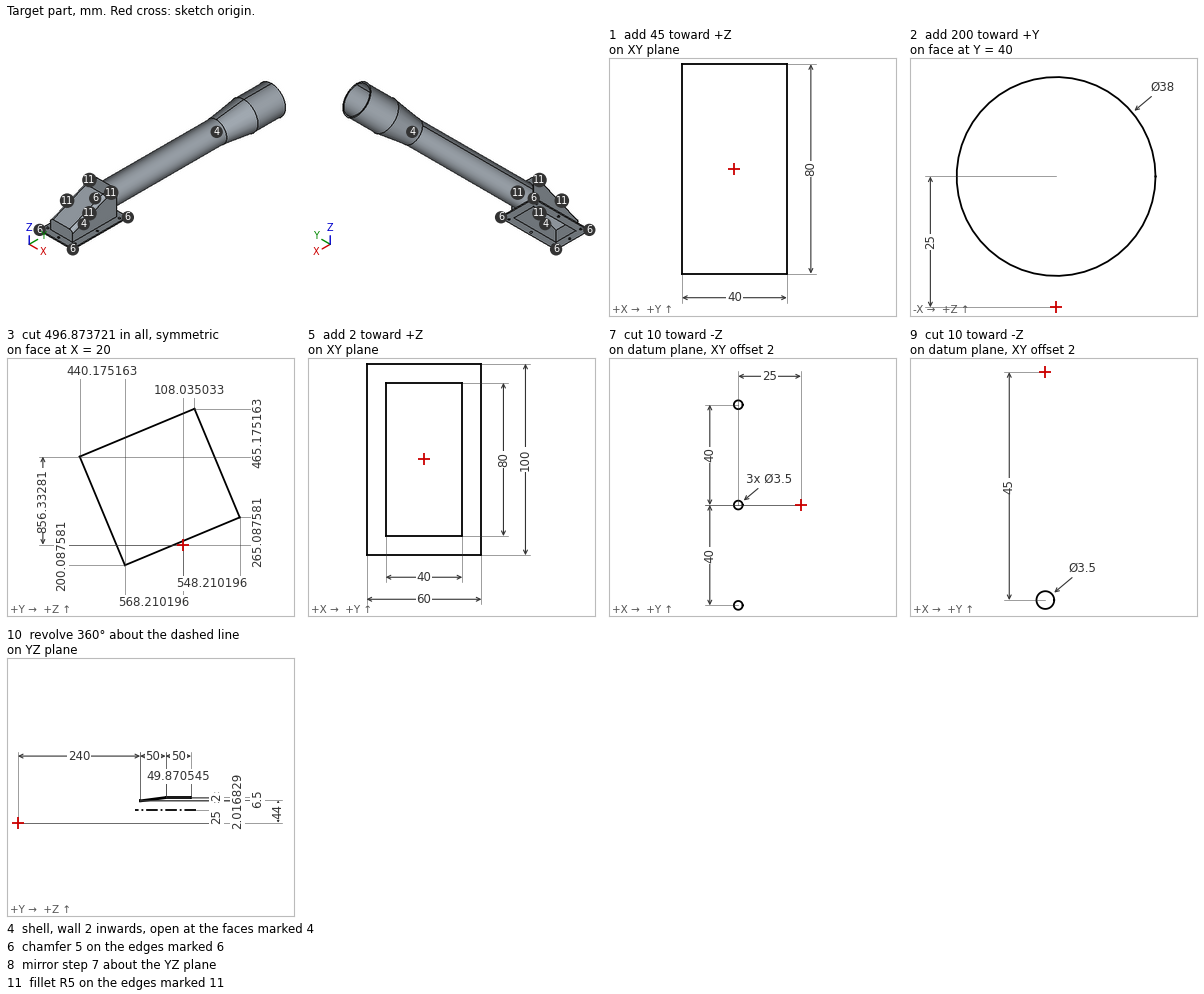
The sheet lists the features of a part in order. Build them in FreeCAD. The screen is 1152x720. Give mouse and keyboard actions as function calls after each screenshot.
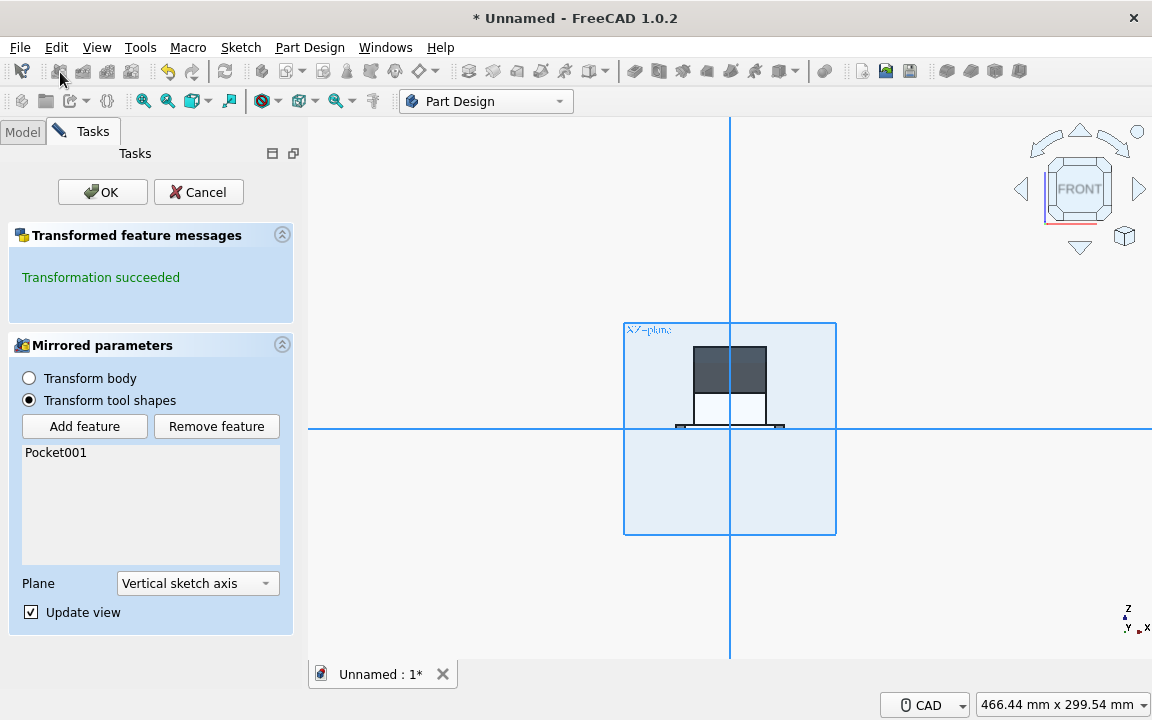
click(198, 584)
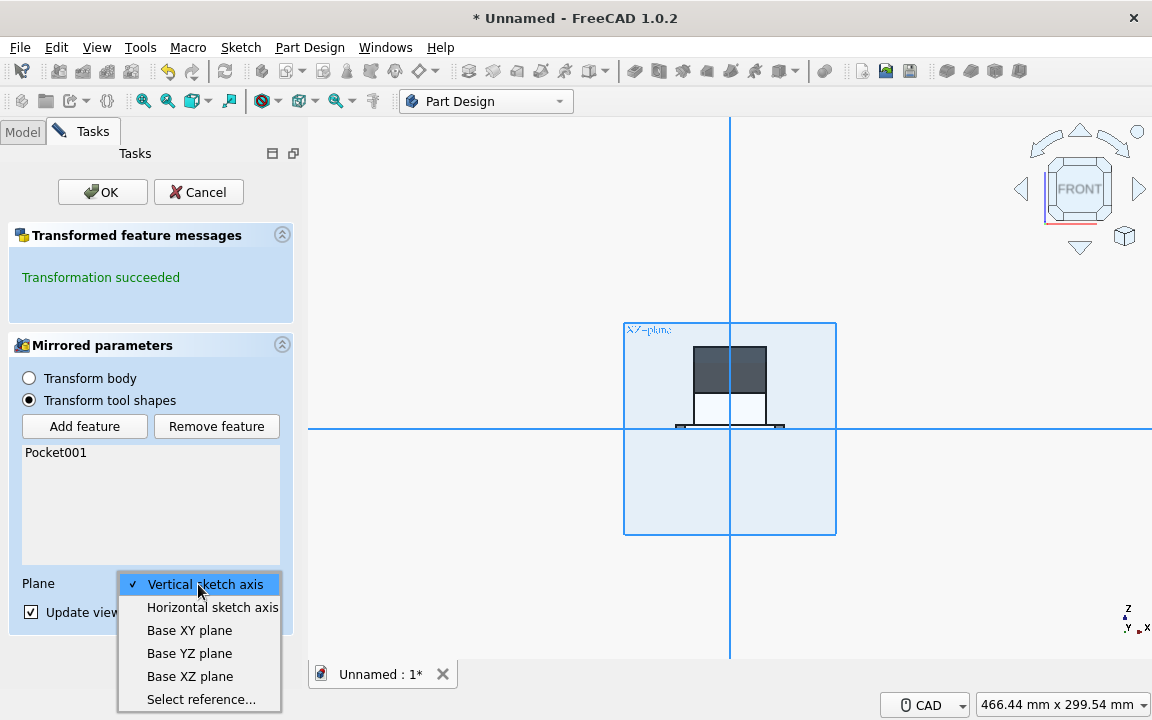
click(198, 654)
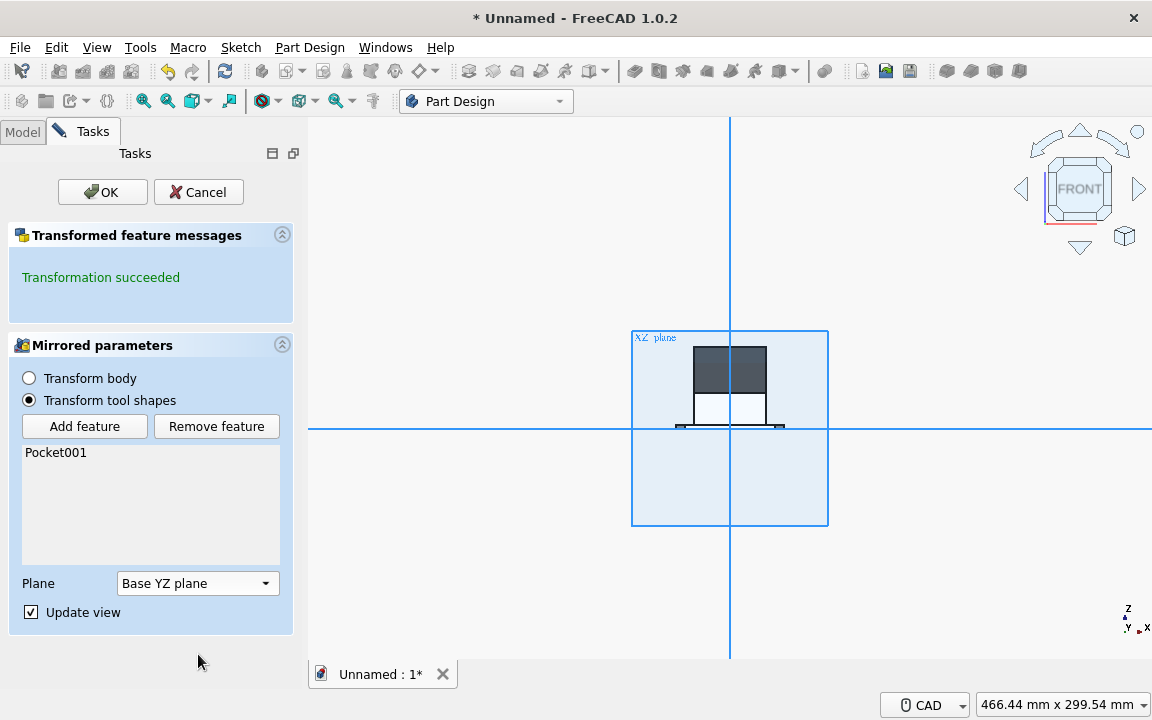
click(103, 192)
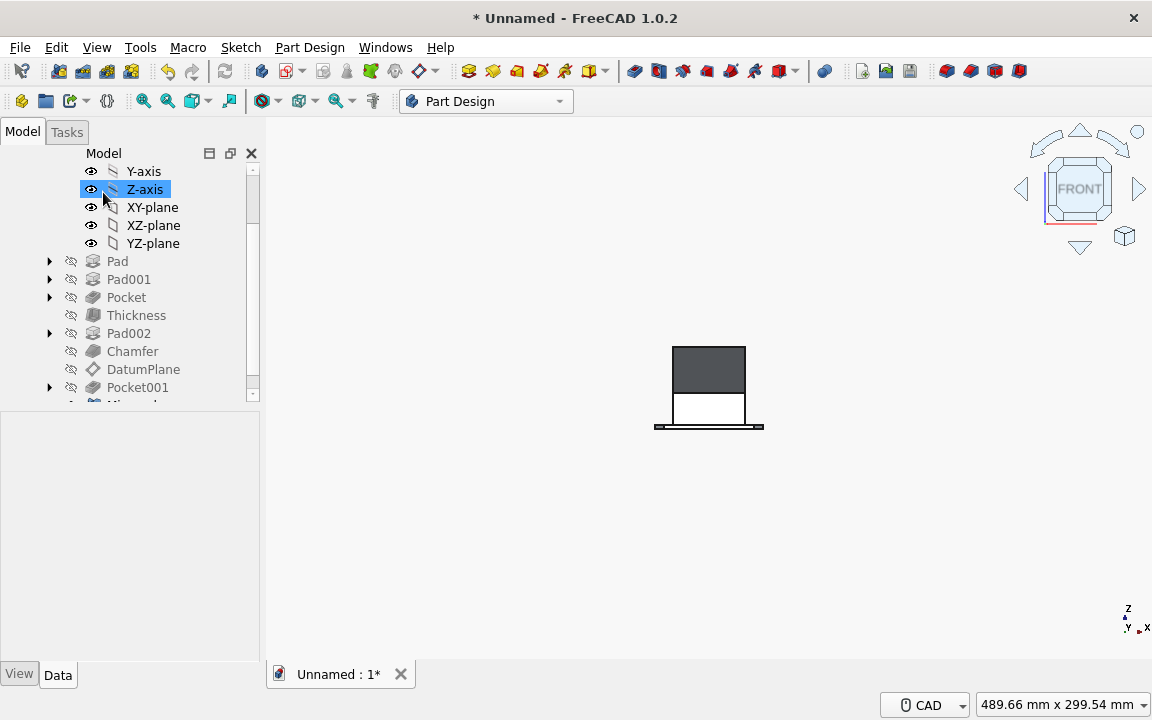
key(v)
key(f)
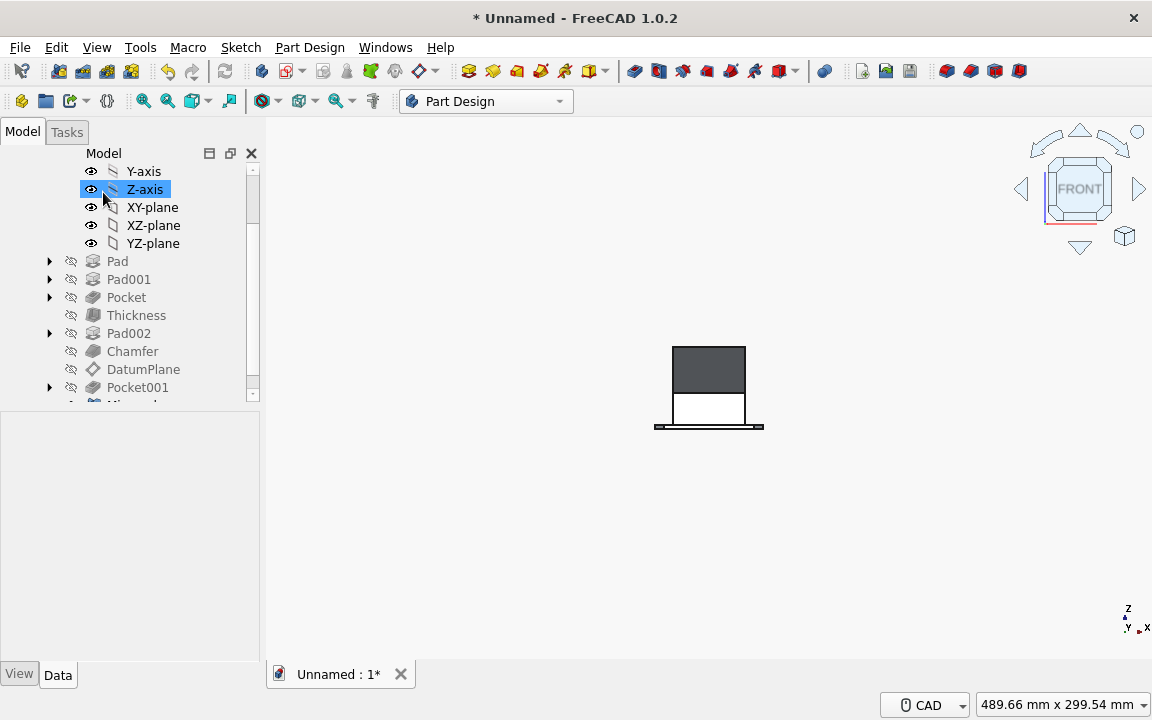
key(0)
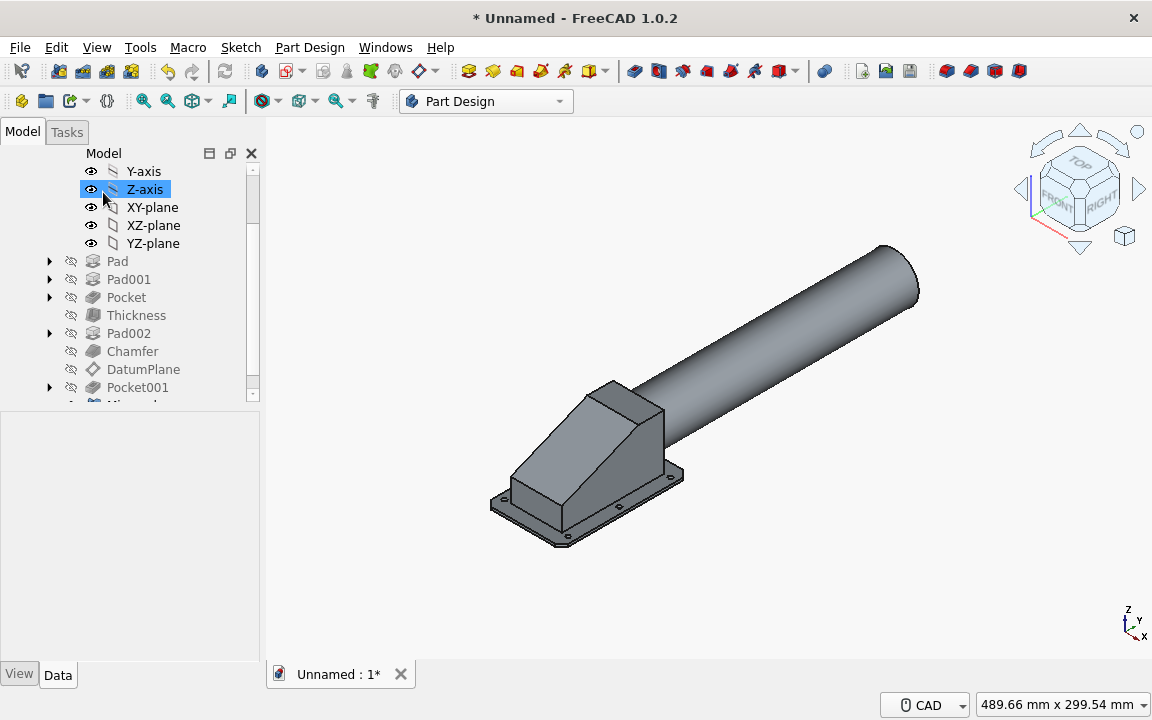
key(2)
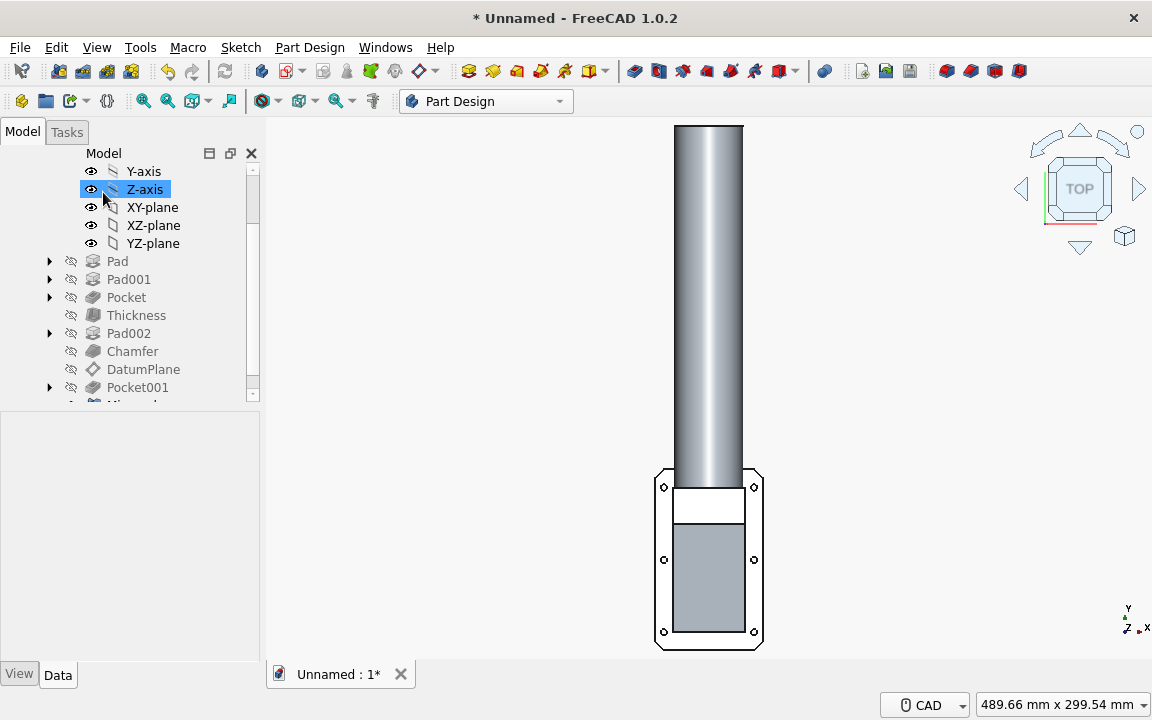
key(1)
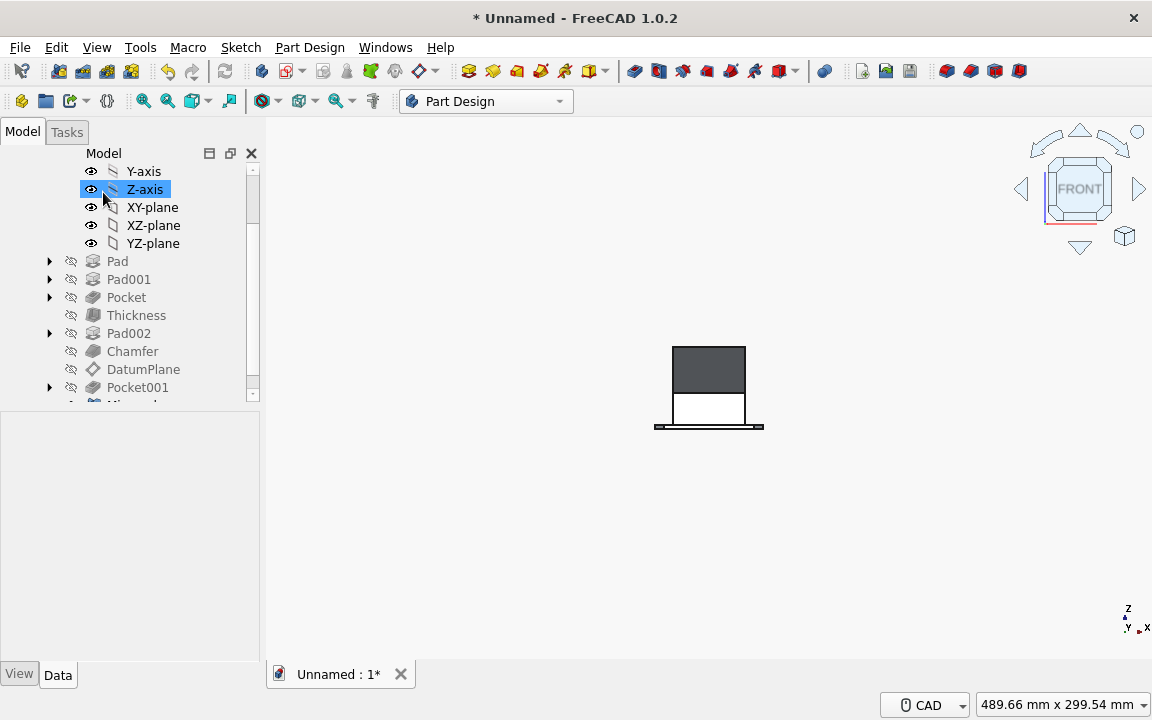
key(v)
key(f)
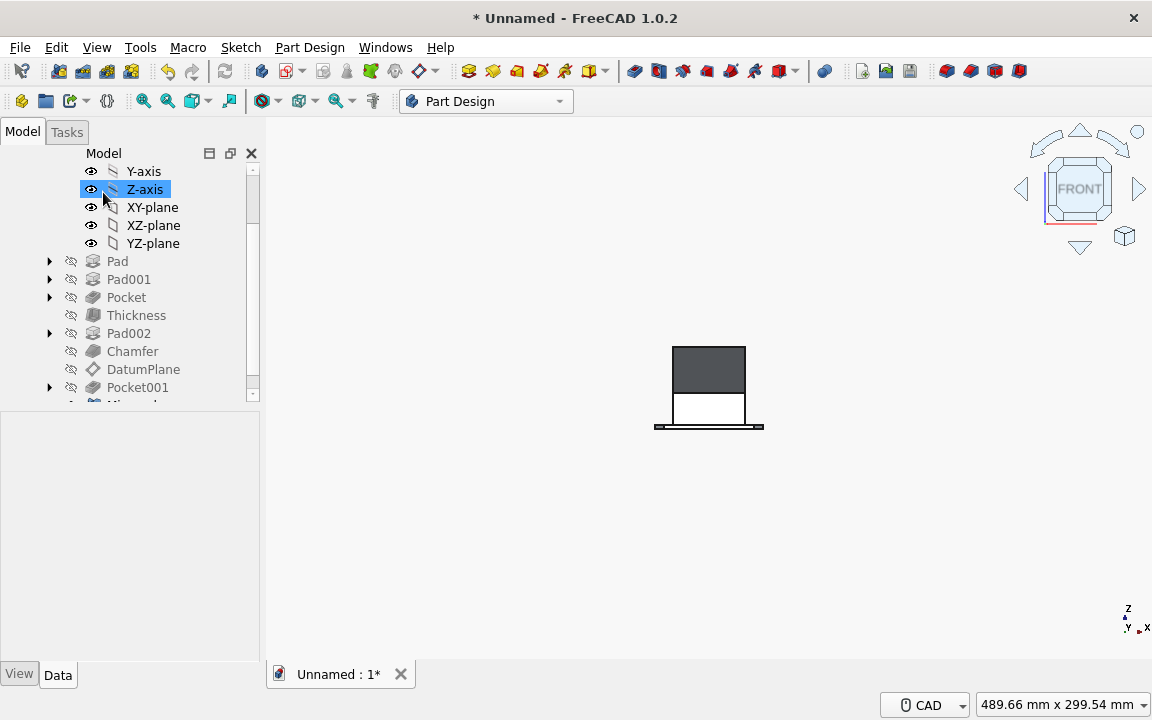
scroll(160, 275, down, 3)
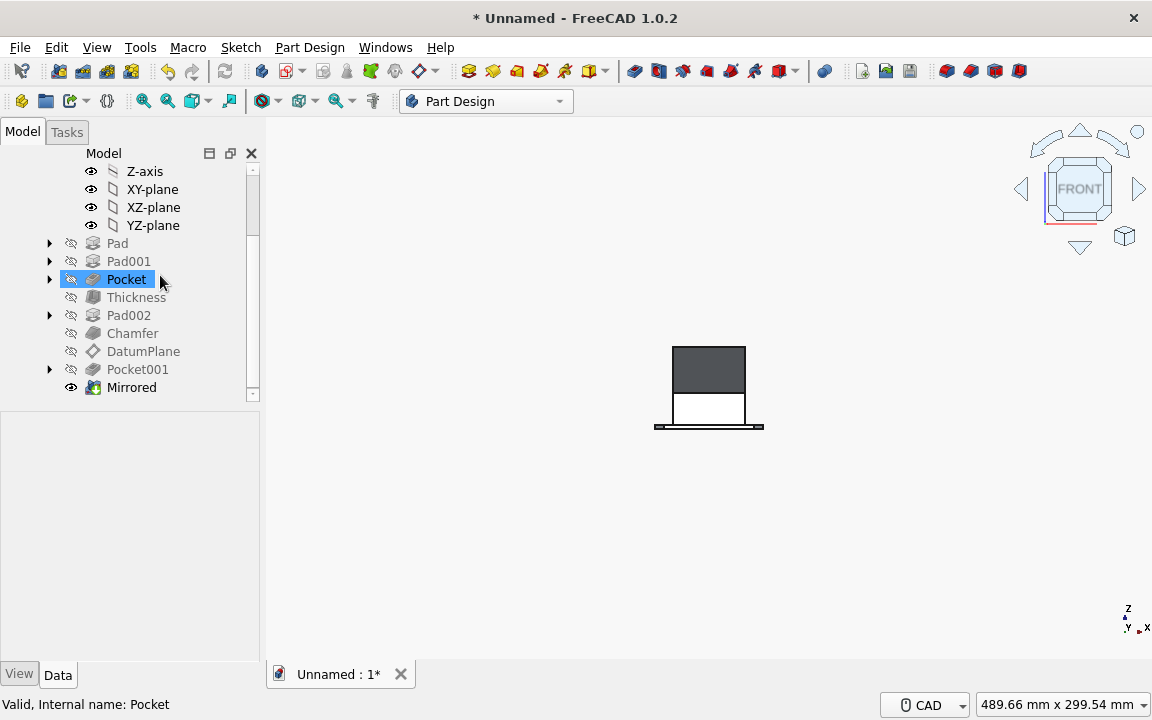
scroll(160, 275, up, 15)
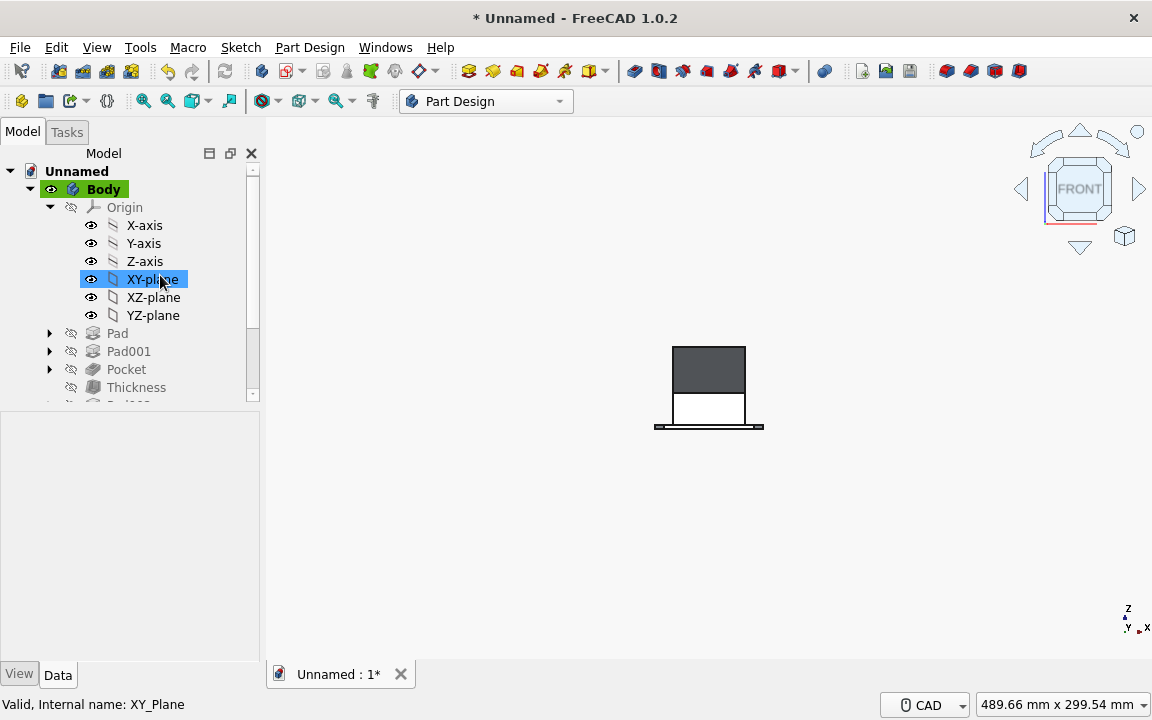
click(136, 279)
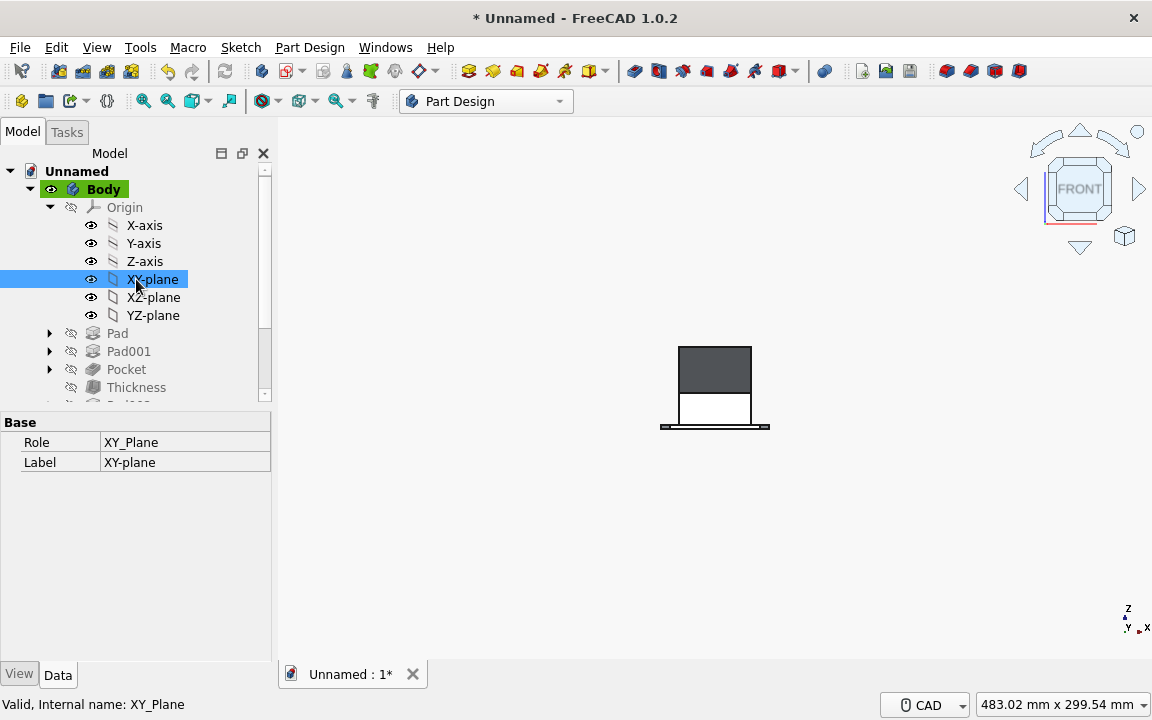
click(420, 72)